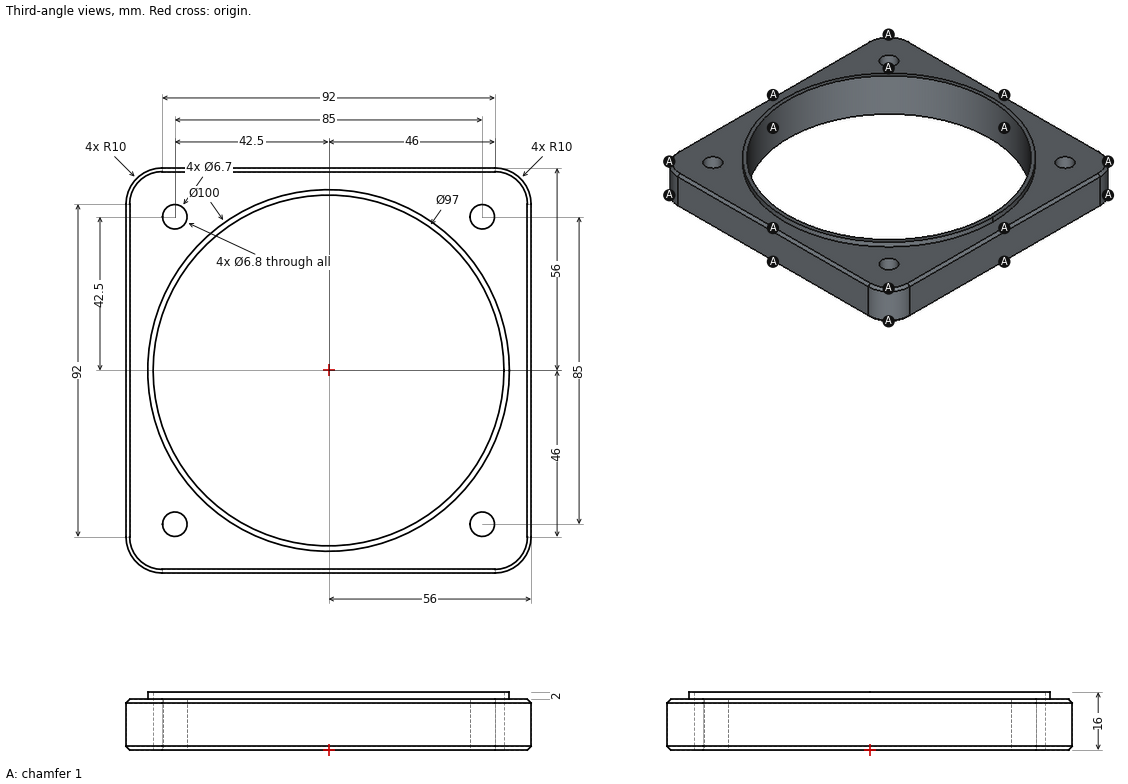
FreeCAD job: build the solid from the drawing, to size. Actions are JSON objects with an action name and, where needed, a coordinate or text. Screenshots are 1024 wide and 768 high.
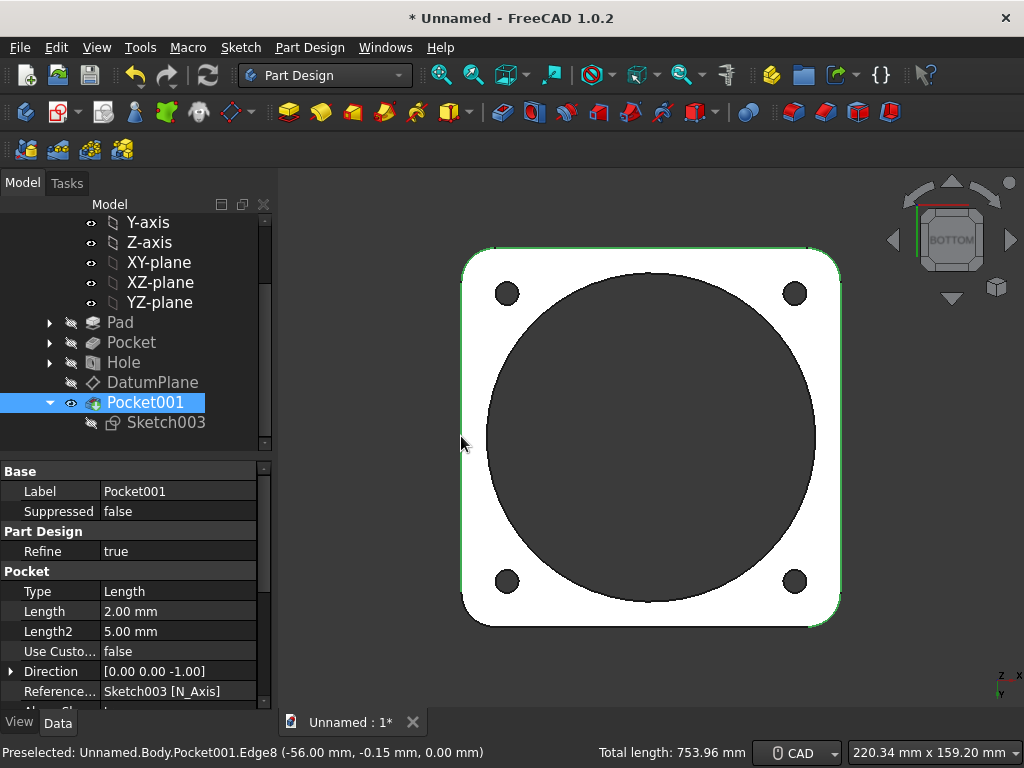
{"action": "left_click", "coordinate": [471, 616], "text": "ctrl"}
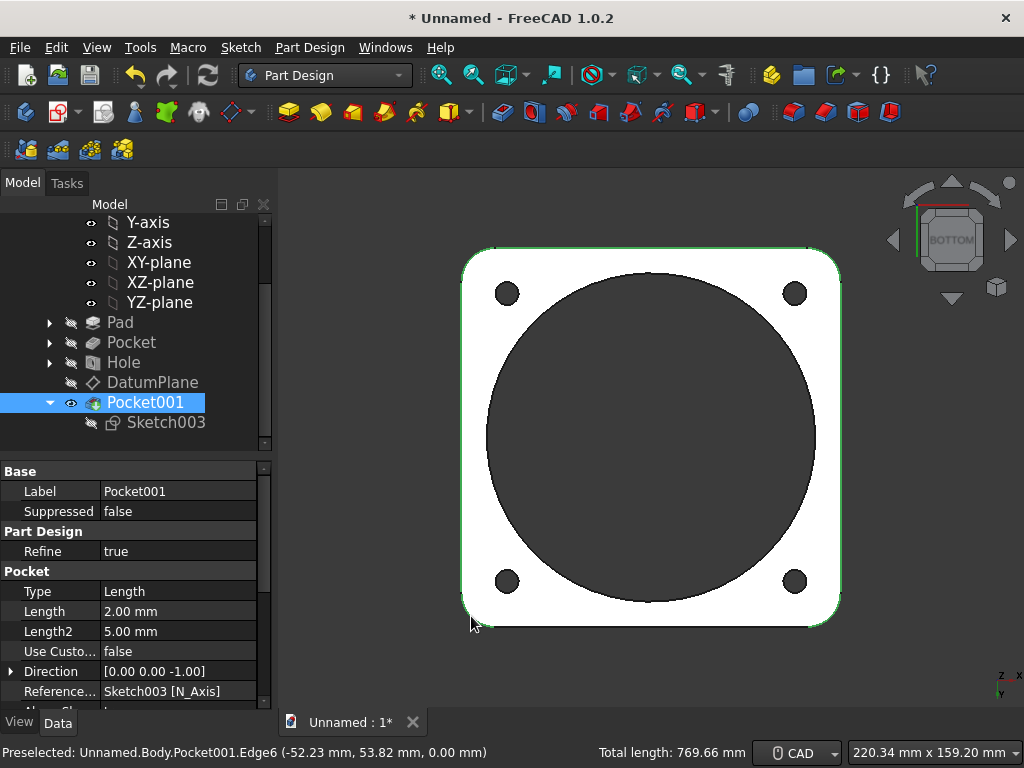
{"action": "left_click", "coordinate": [651, 626], "text": "ctrl"}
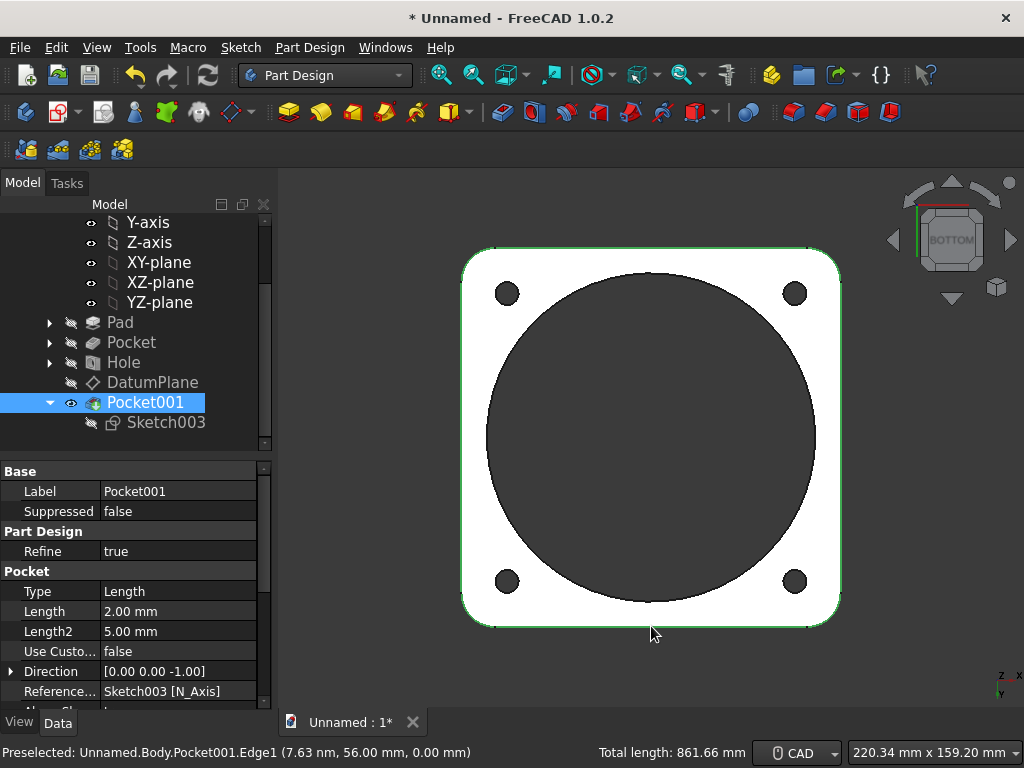
{"action": "left_click", "coordinate": [826, 112]}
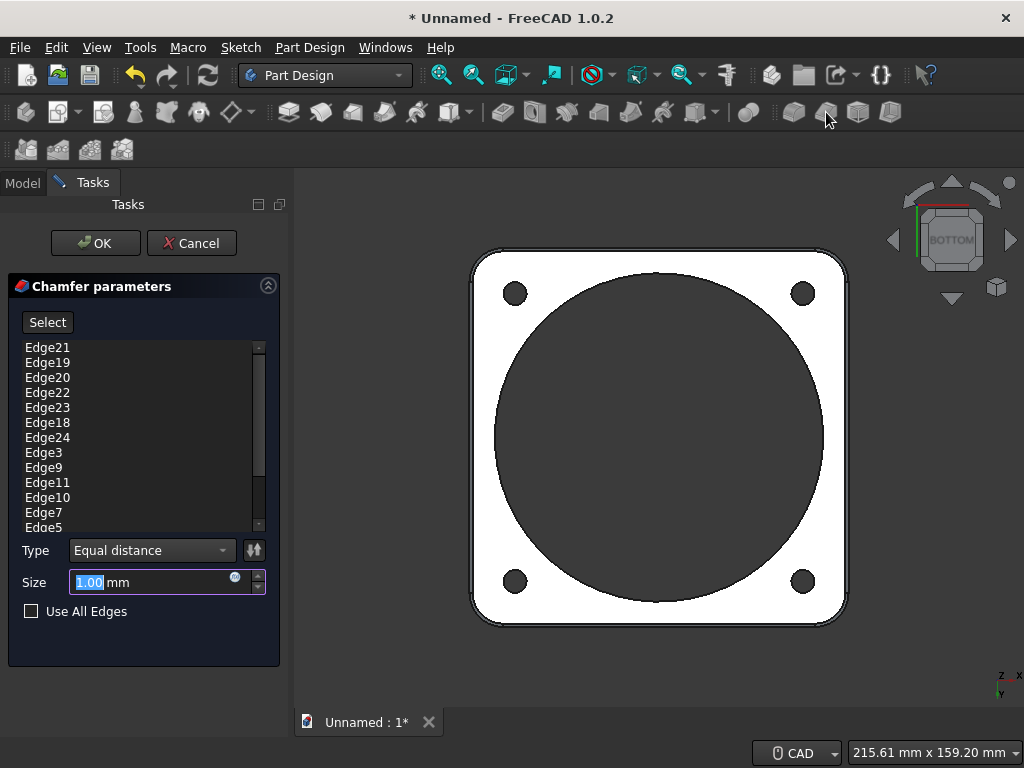
{"action": "type", "text": "1"}
{"action": "key", "text": "Tab"}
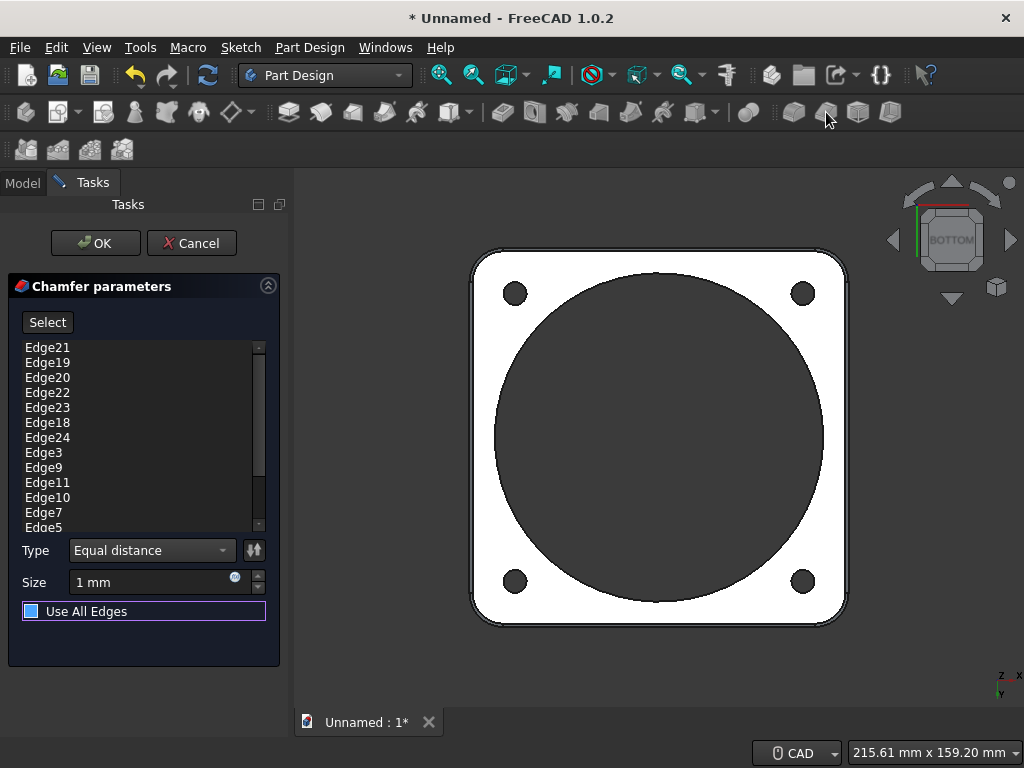
{"action": "left_click", "coordinate": [96, 243]}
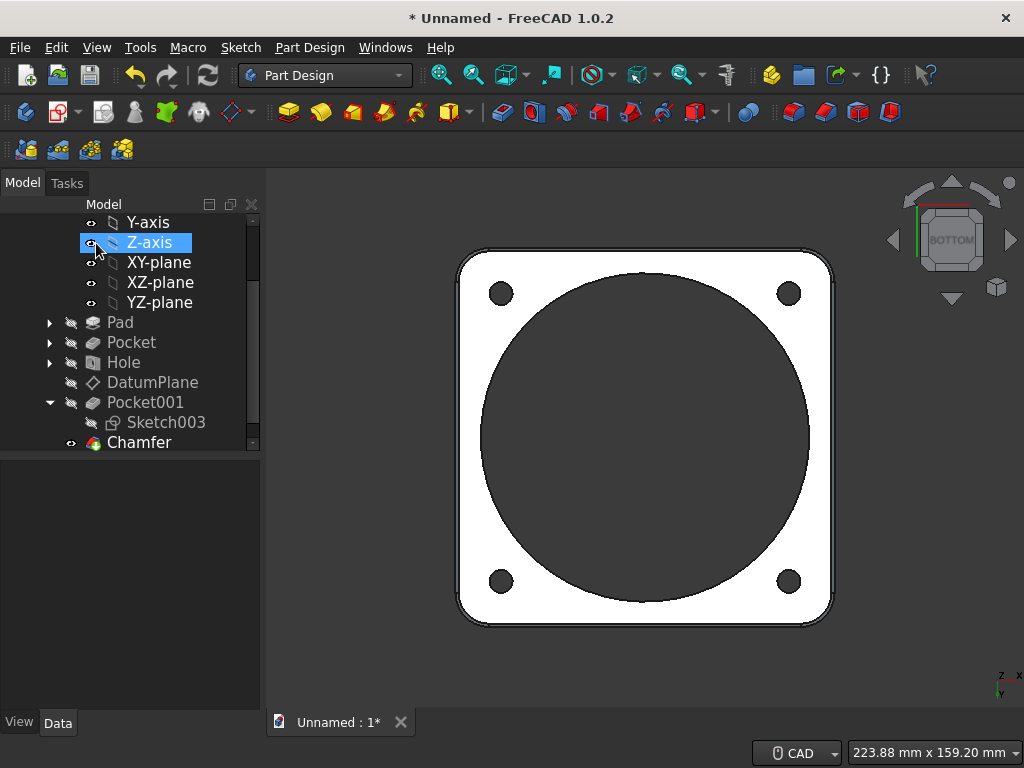
{"action": "key", "text": "0"}